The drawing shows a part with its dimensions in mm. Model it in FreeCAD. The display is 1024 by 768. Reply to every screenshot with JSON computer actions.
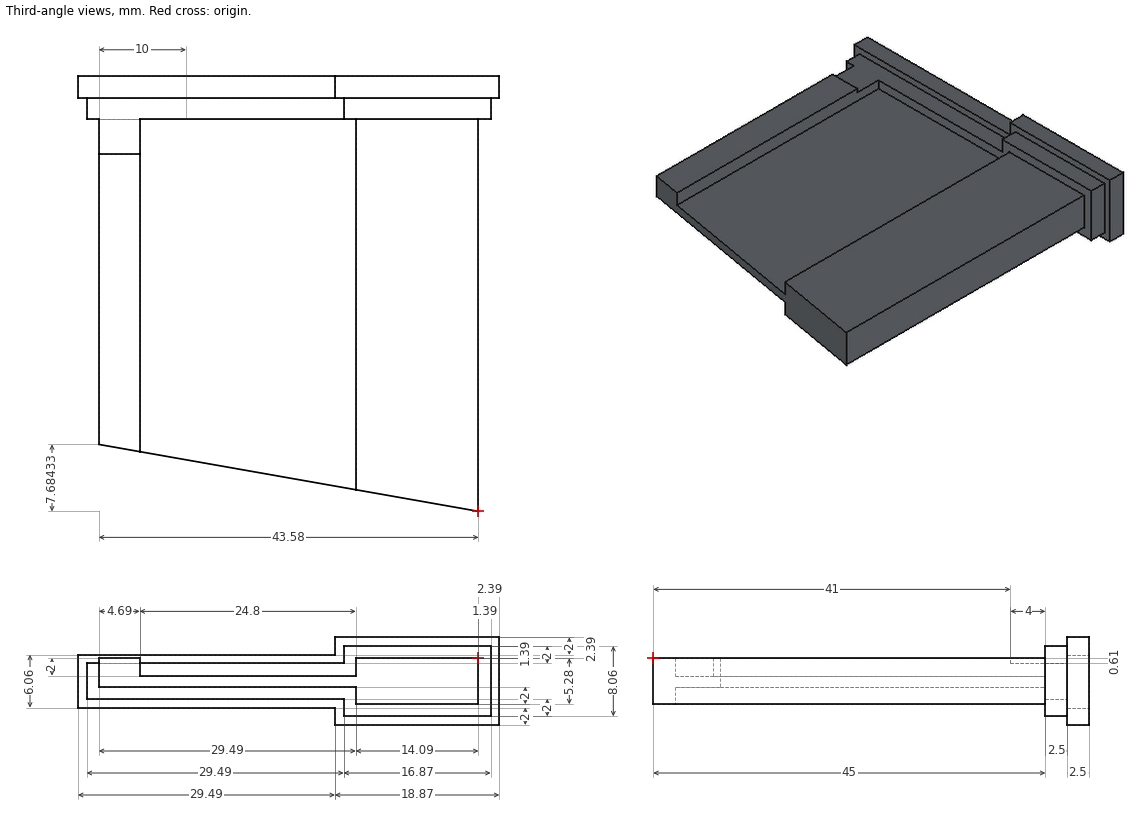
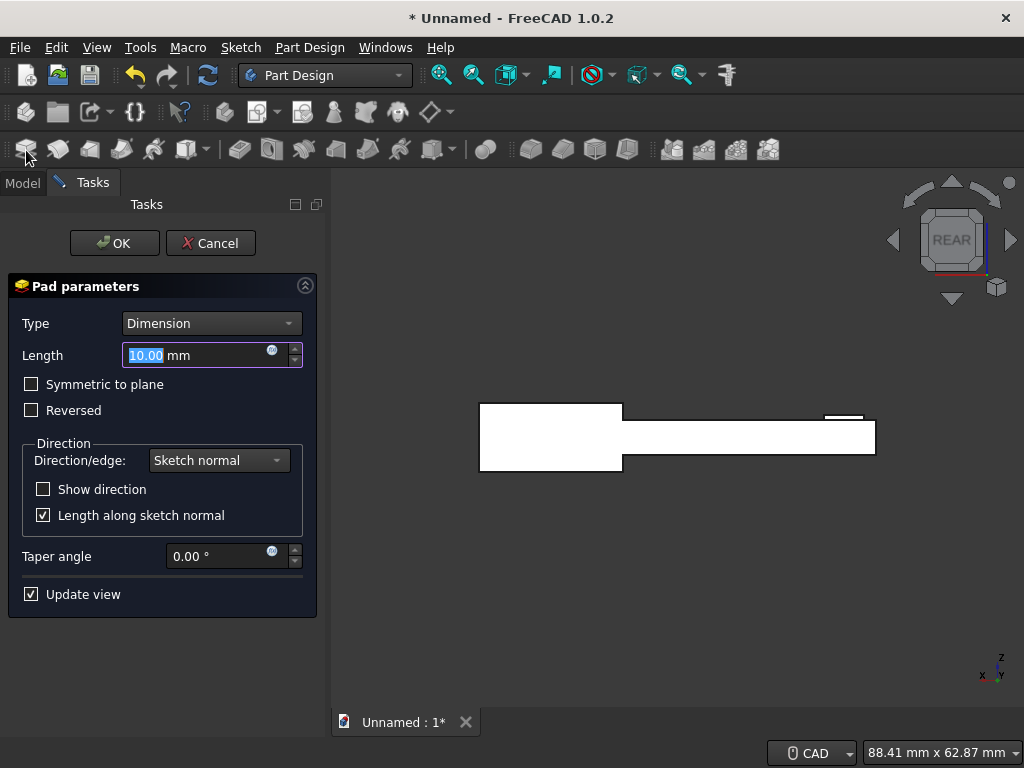
{"action": "type", "text": "2.5"}
{"action": "key", "text": "Tab"}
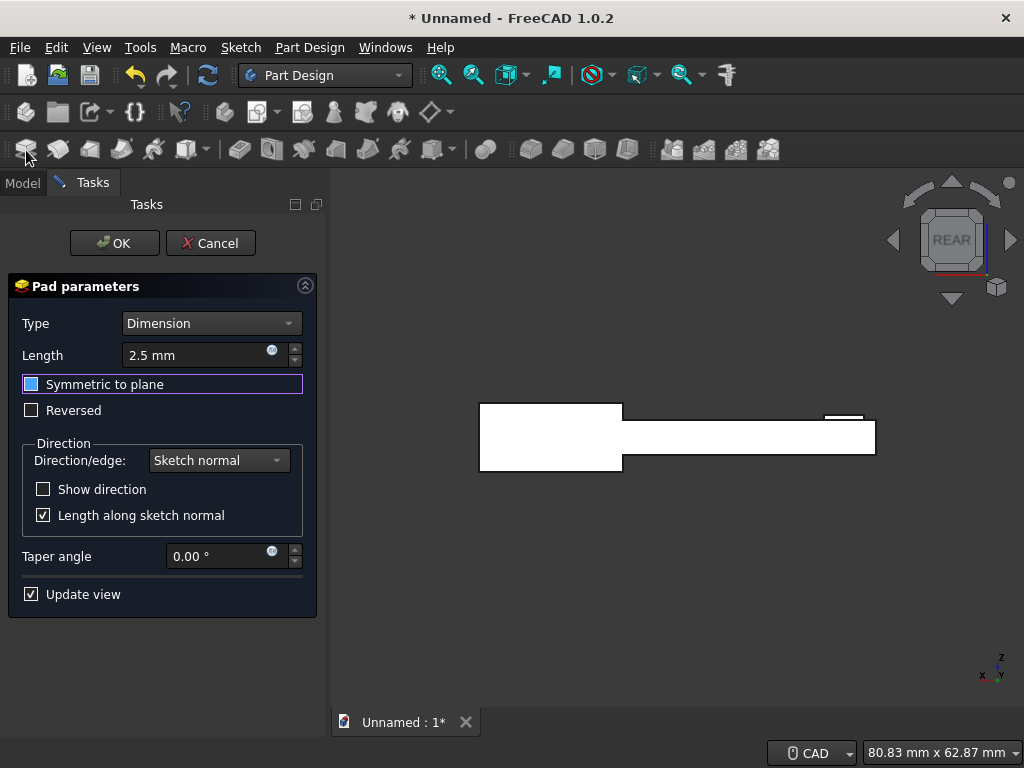
{"action": "left_click", "coordinate": [115, 243]}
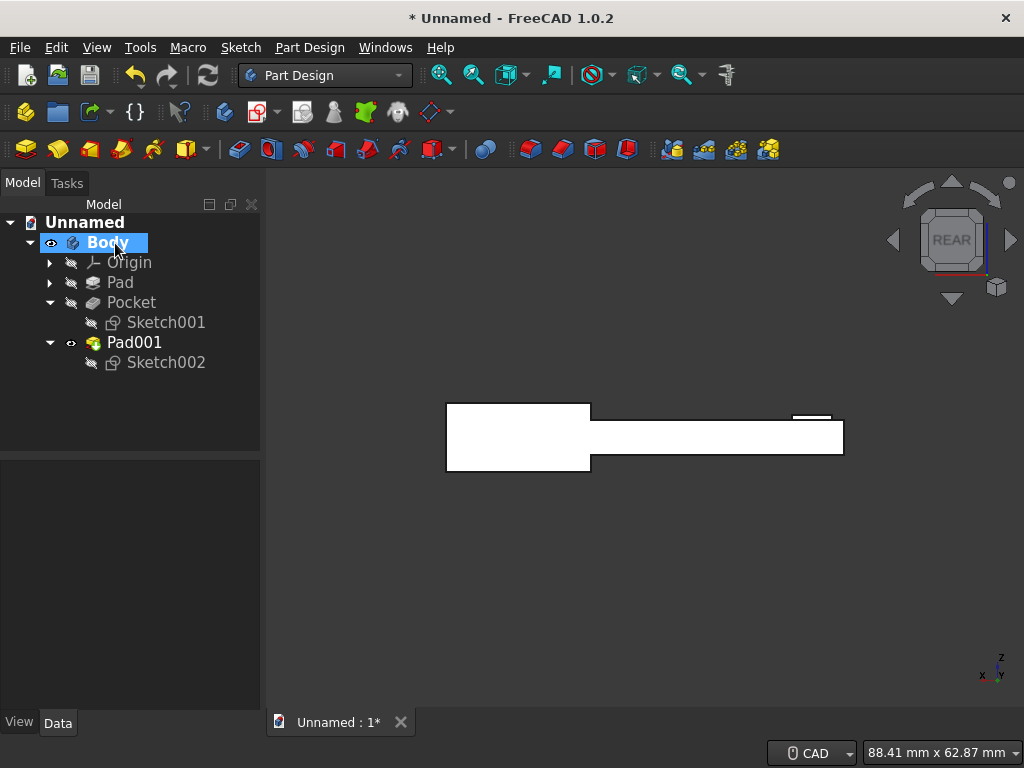
{"action": "left_click", "coordinate": [531, 437]}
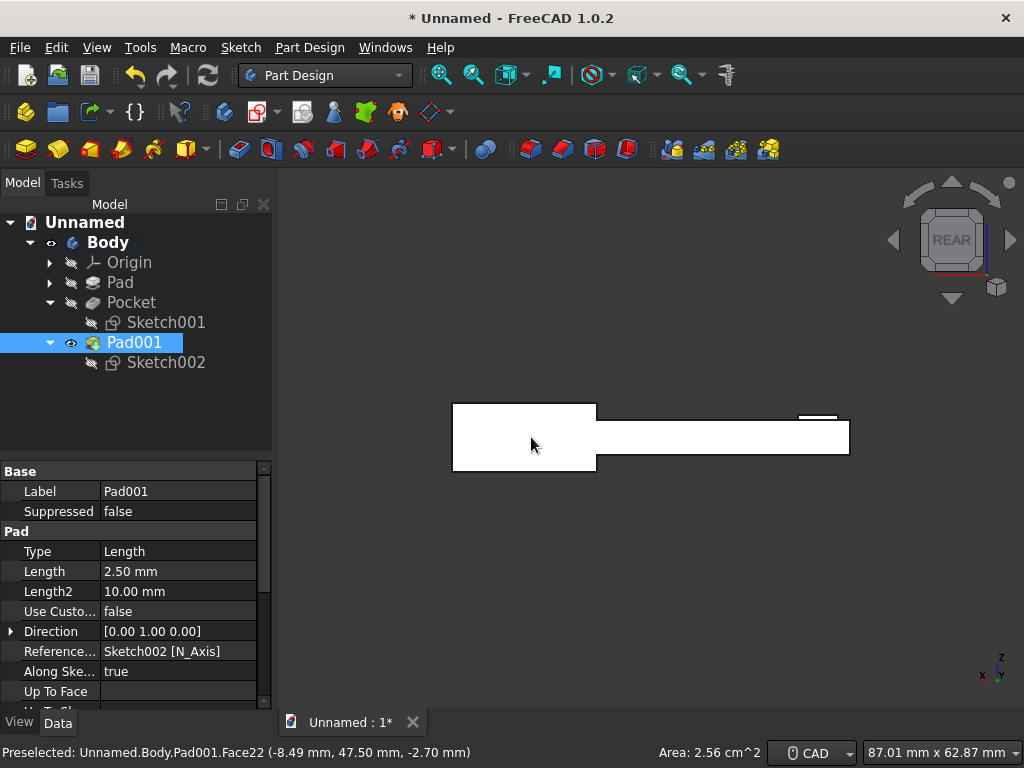
{"action": "left_click", "coordinate": [258, 112]}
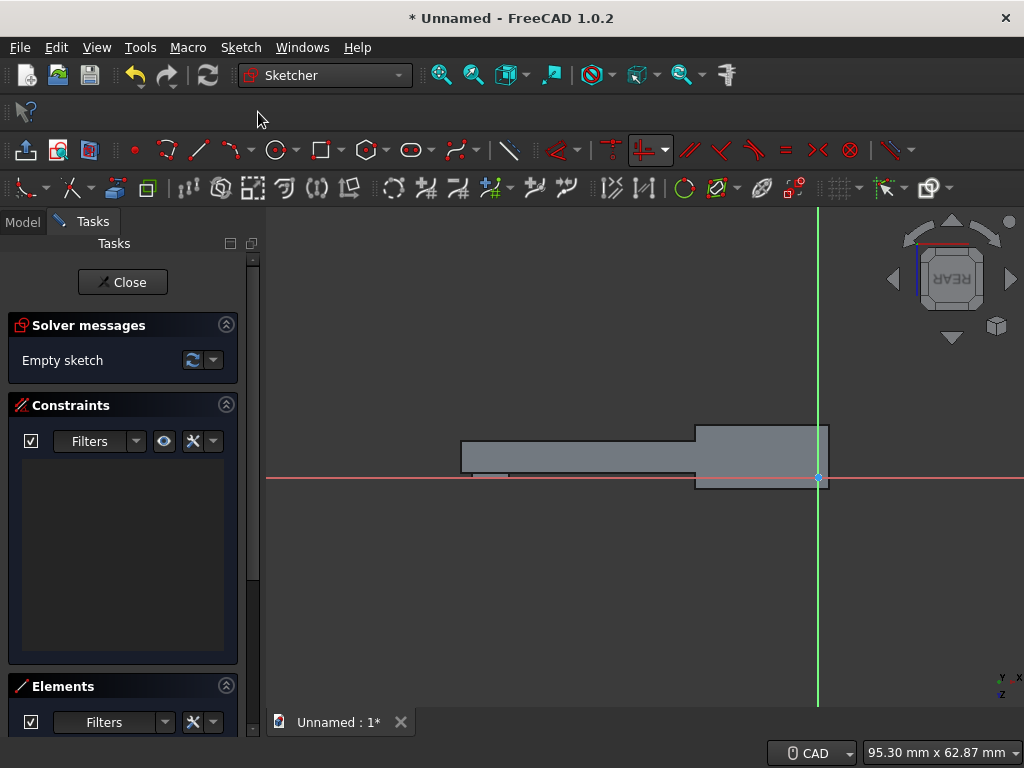
{"action": "scroll", "coordinate": [294, 457], "scroll_direction": "down", "scroll_amount": 1}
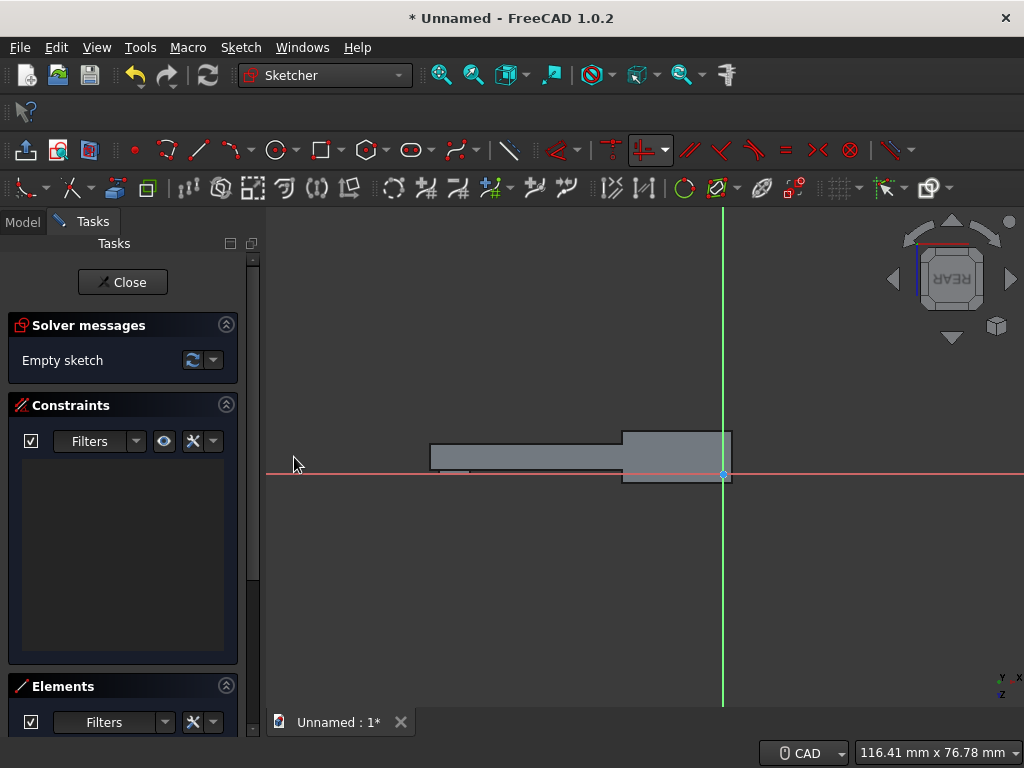
{"action": "key", "text": "g m"}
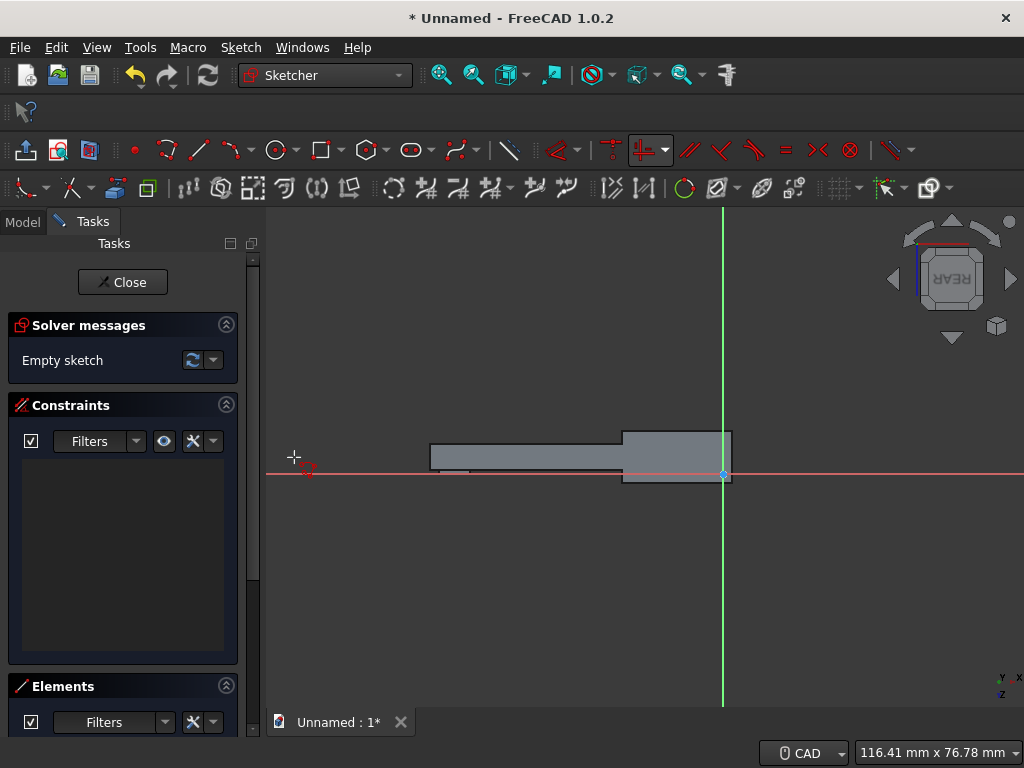
{"action": "left_click", "coordinate": [739, 490]}
{"action": "left_click", "coordinate": [739, 424]}
{"action": "left_click", "coordinate": [616, 424]}
{"action": "left_click", "coordinate": [616, 437]}
{"action": "left_click", "coordinate": [424, 437]}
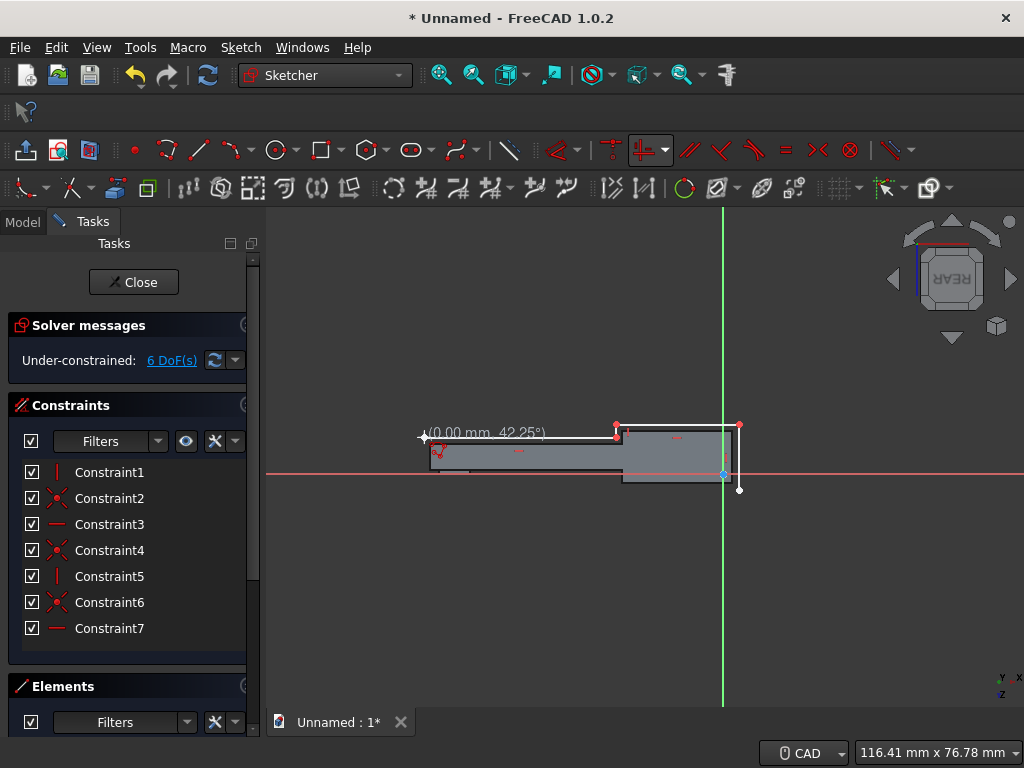
{"action": "scroll", "coordinate": [424, 477], "scroll_direction": "up", "scroll_amount": 10}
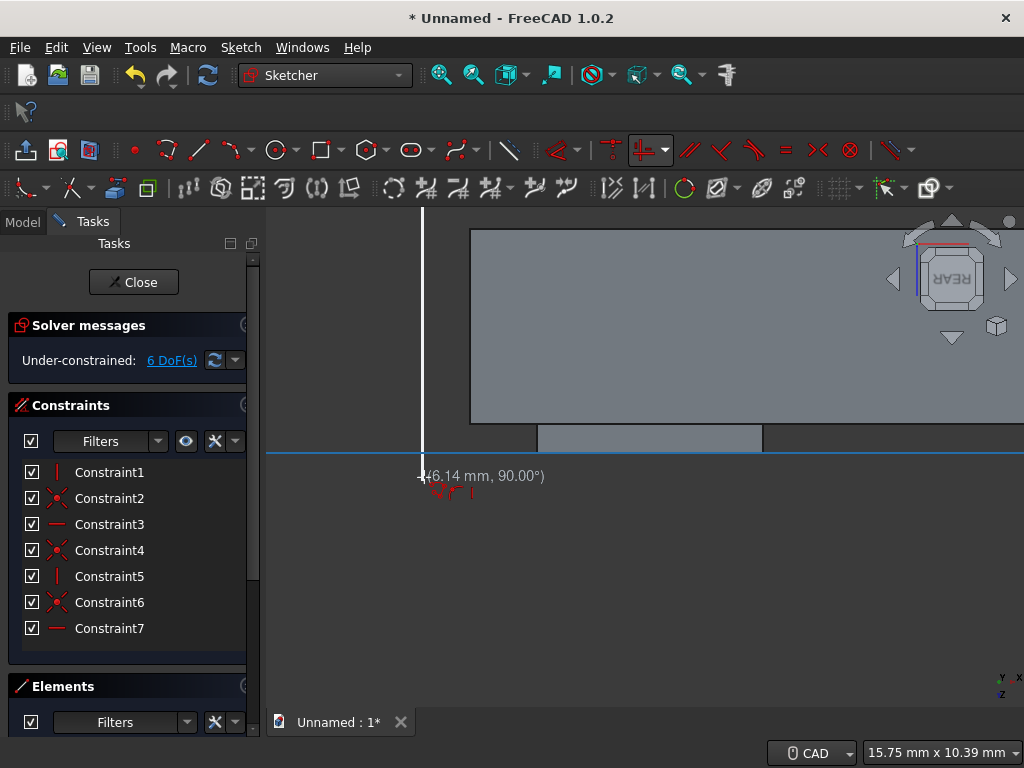
{"action": "left_click", "coordinate": [423, 472]}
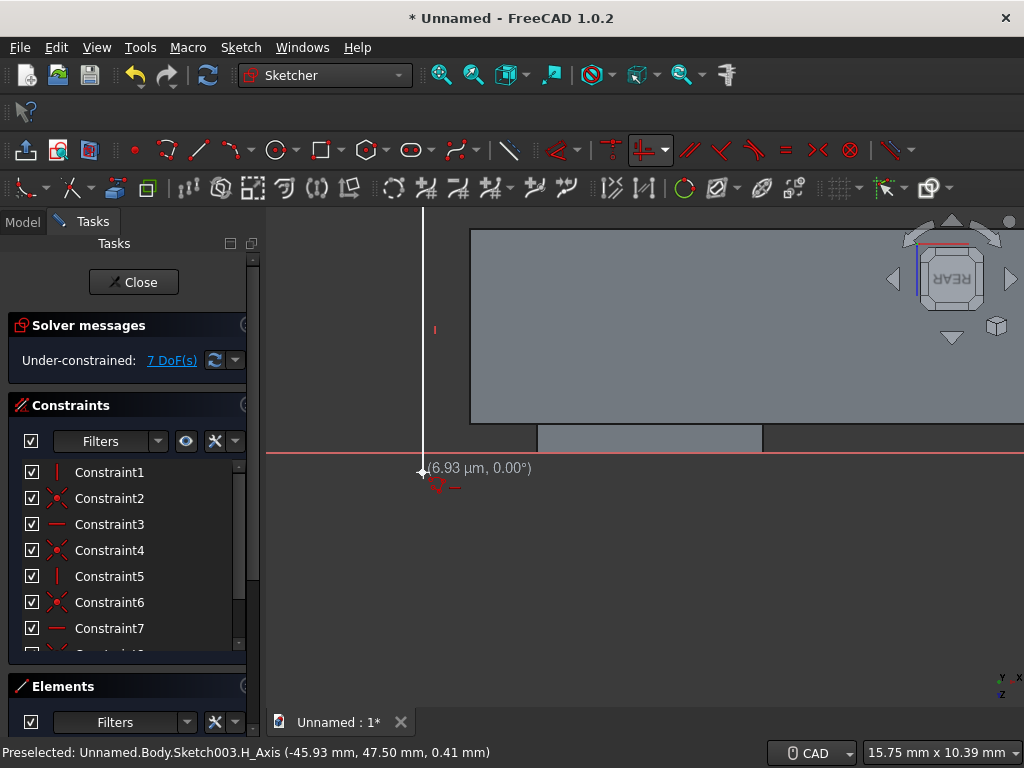
{"action": "scroll", "coordinate": [377, 483], "scroll_direction": "down", "scroll_amount": 9}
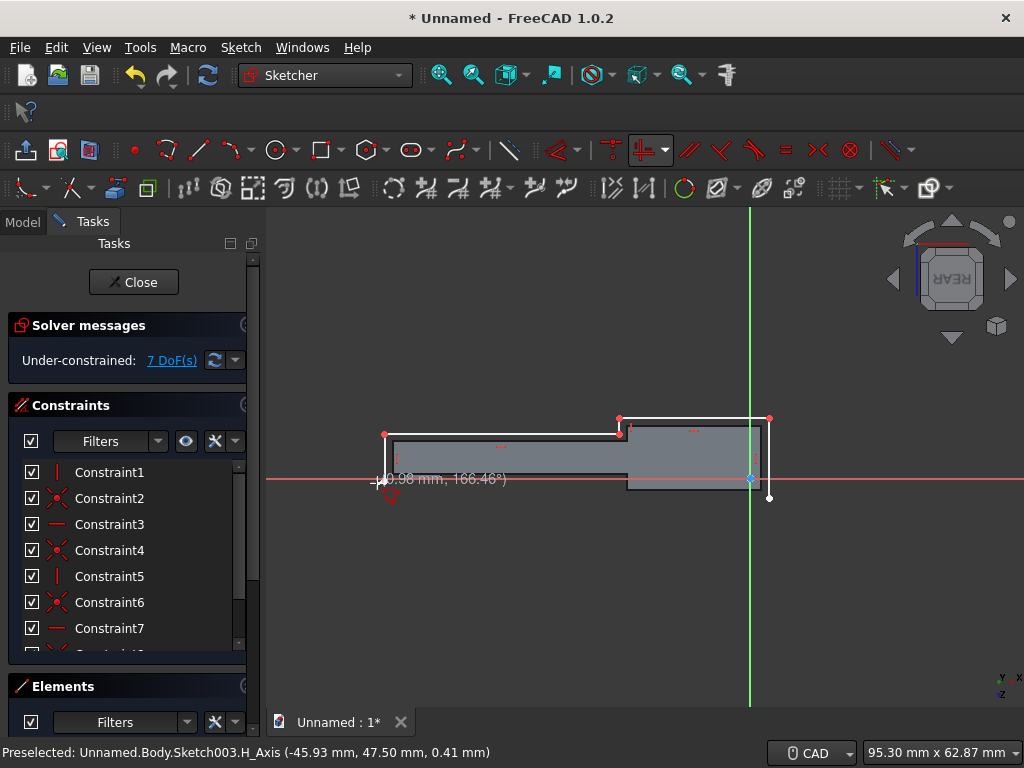
{"action": "scroll", "coordinate": [619, 482], "scroll_direction": "up", "scroll_amount": 9}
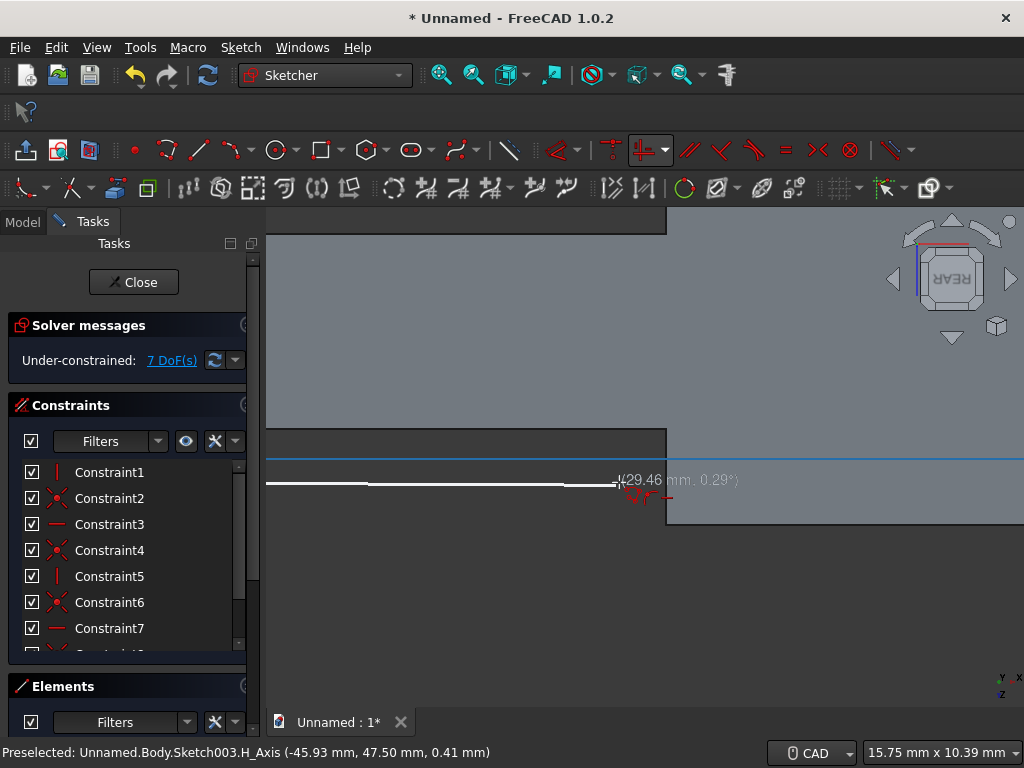
{"action": "left_click", "coordinate": [617, 477]}